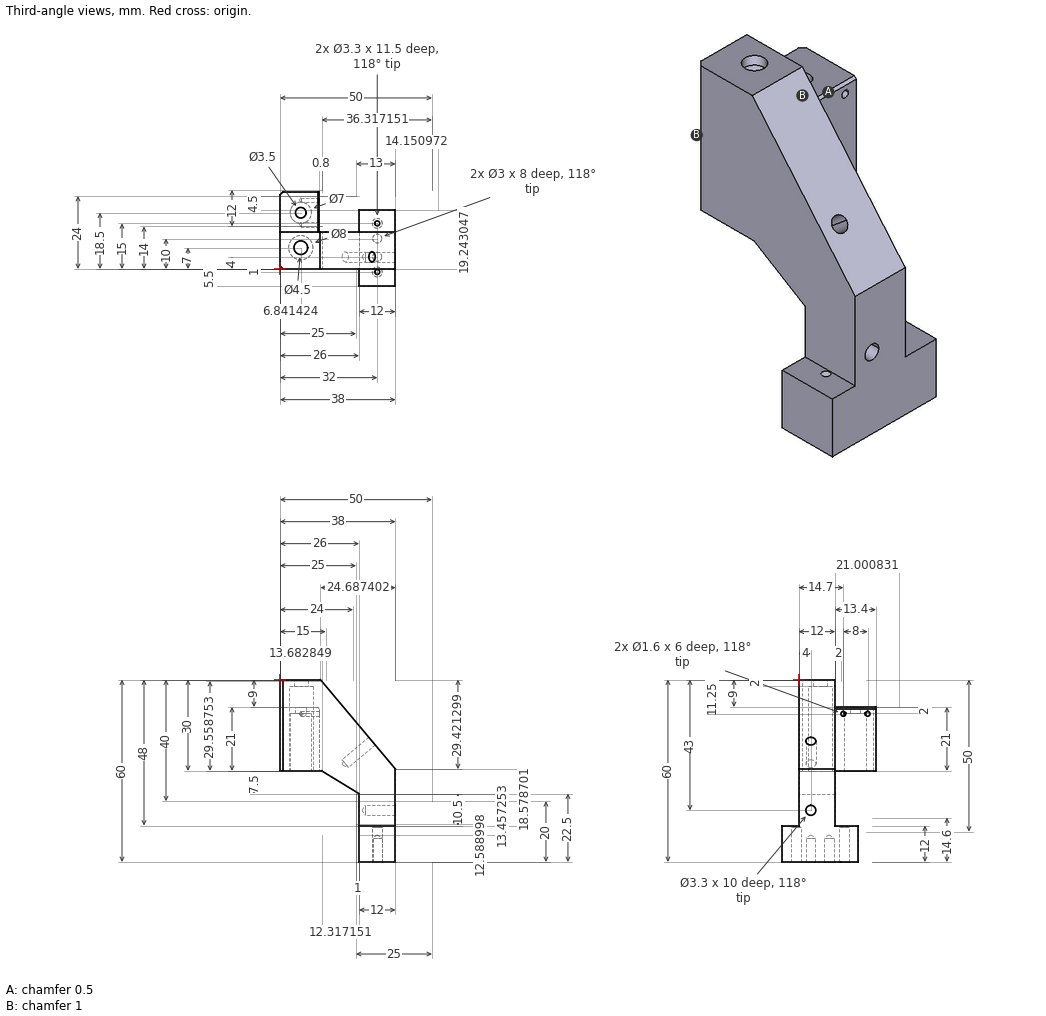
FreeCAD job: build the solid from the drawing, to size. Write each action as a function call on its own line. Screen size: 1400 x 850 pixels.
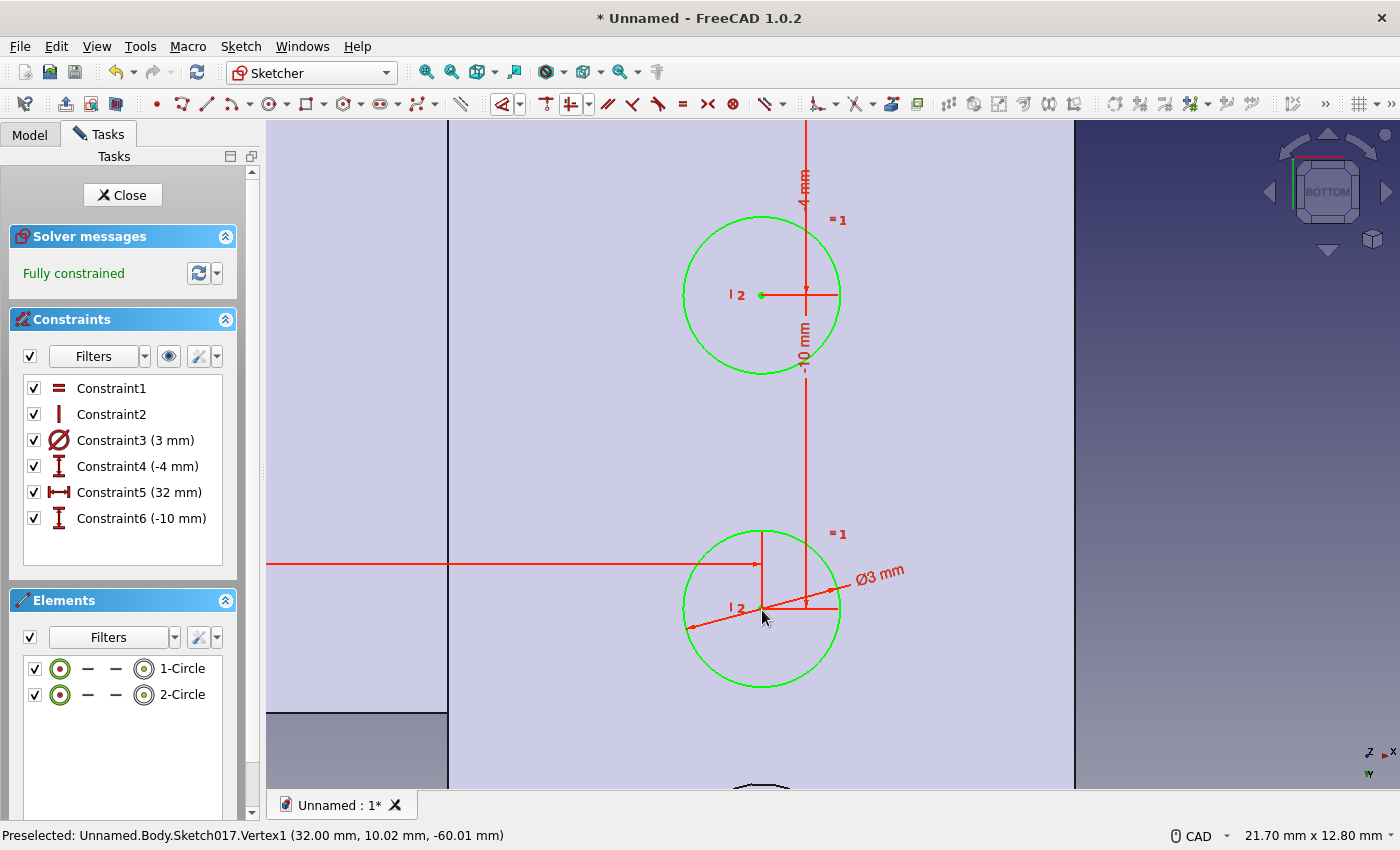
click(123, 195)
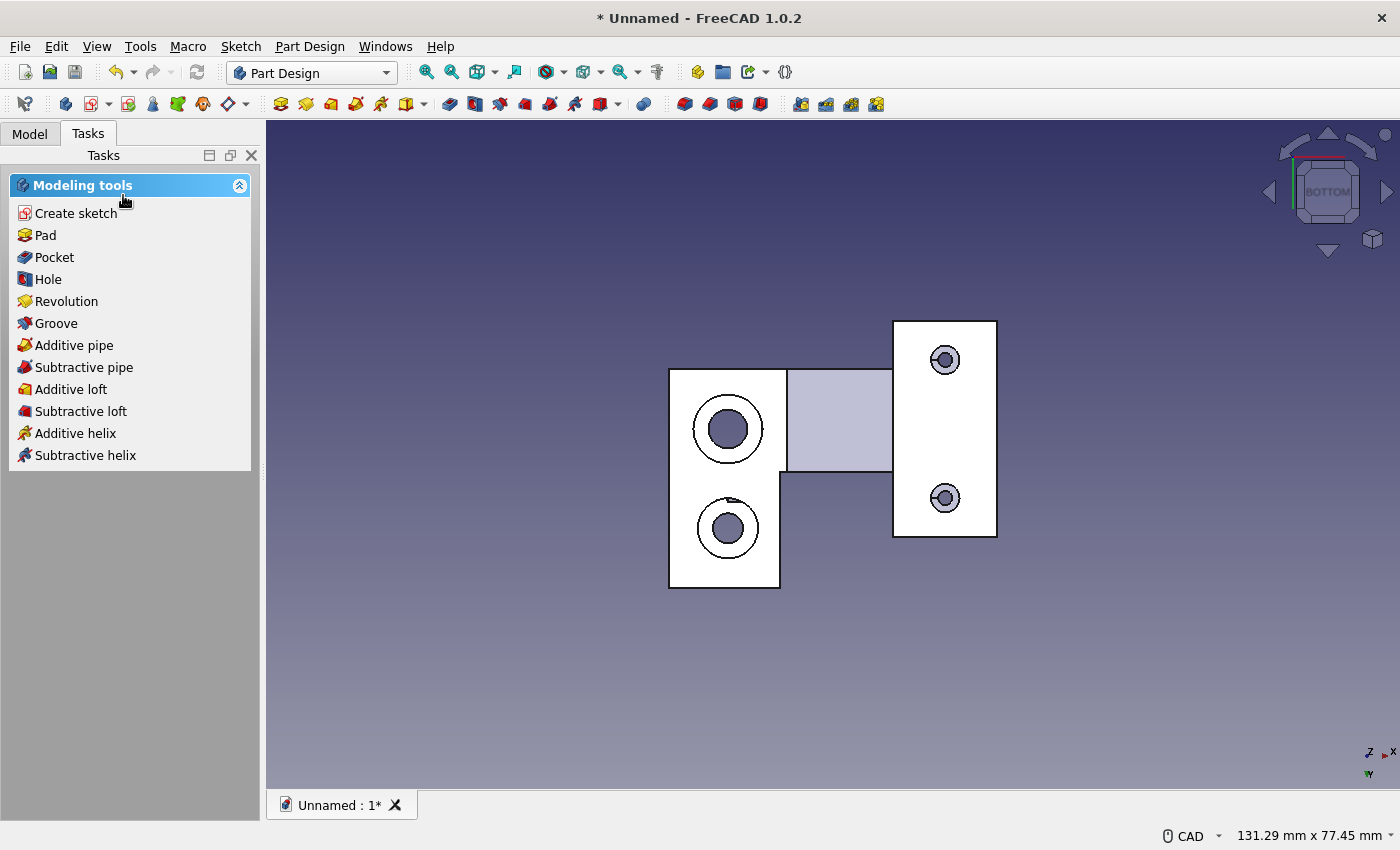
click(475, 104)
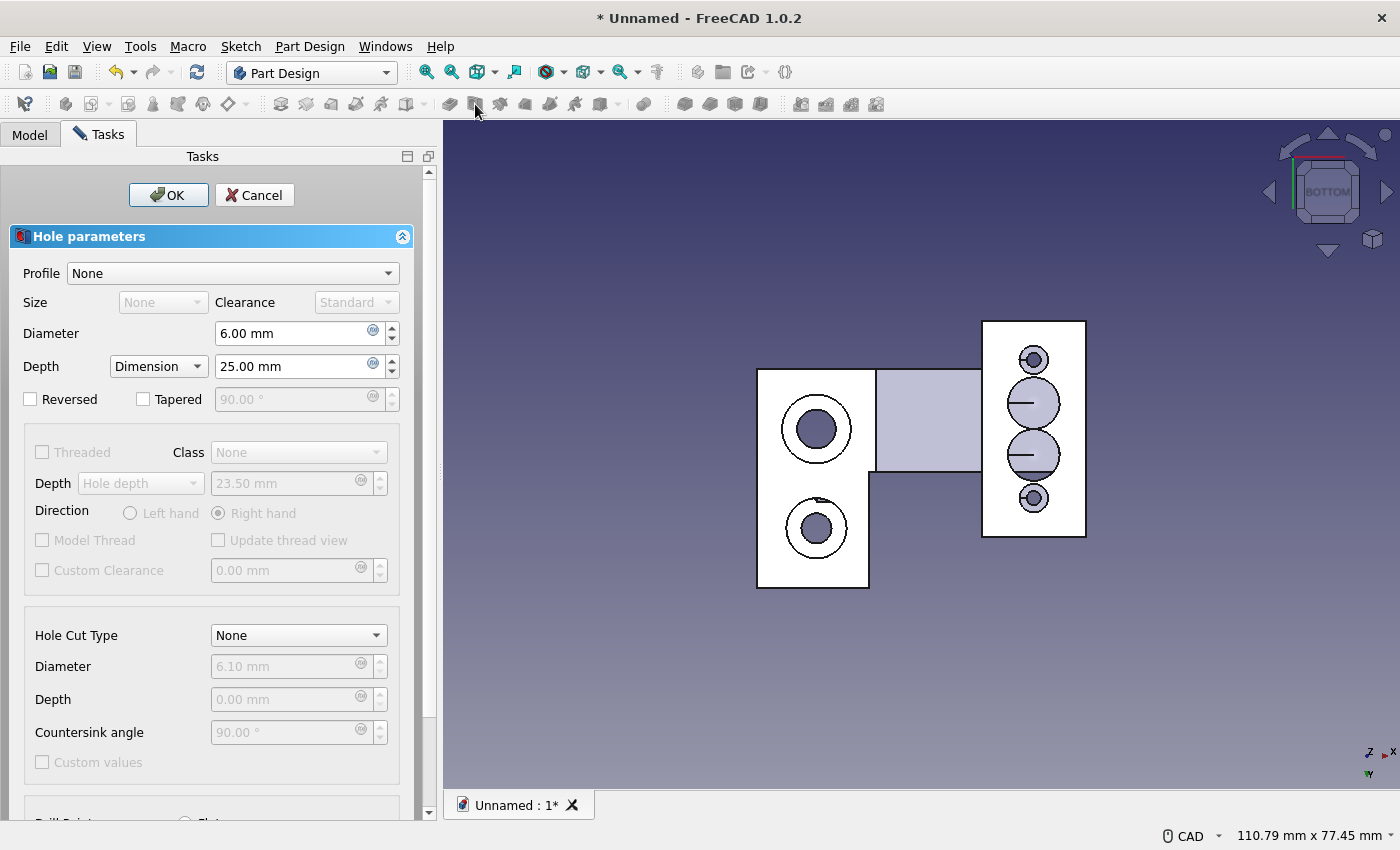
triple_click(300, 334)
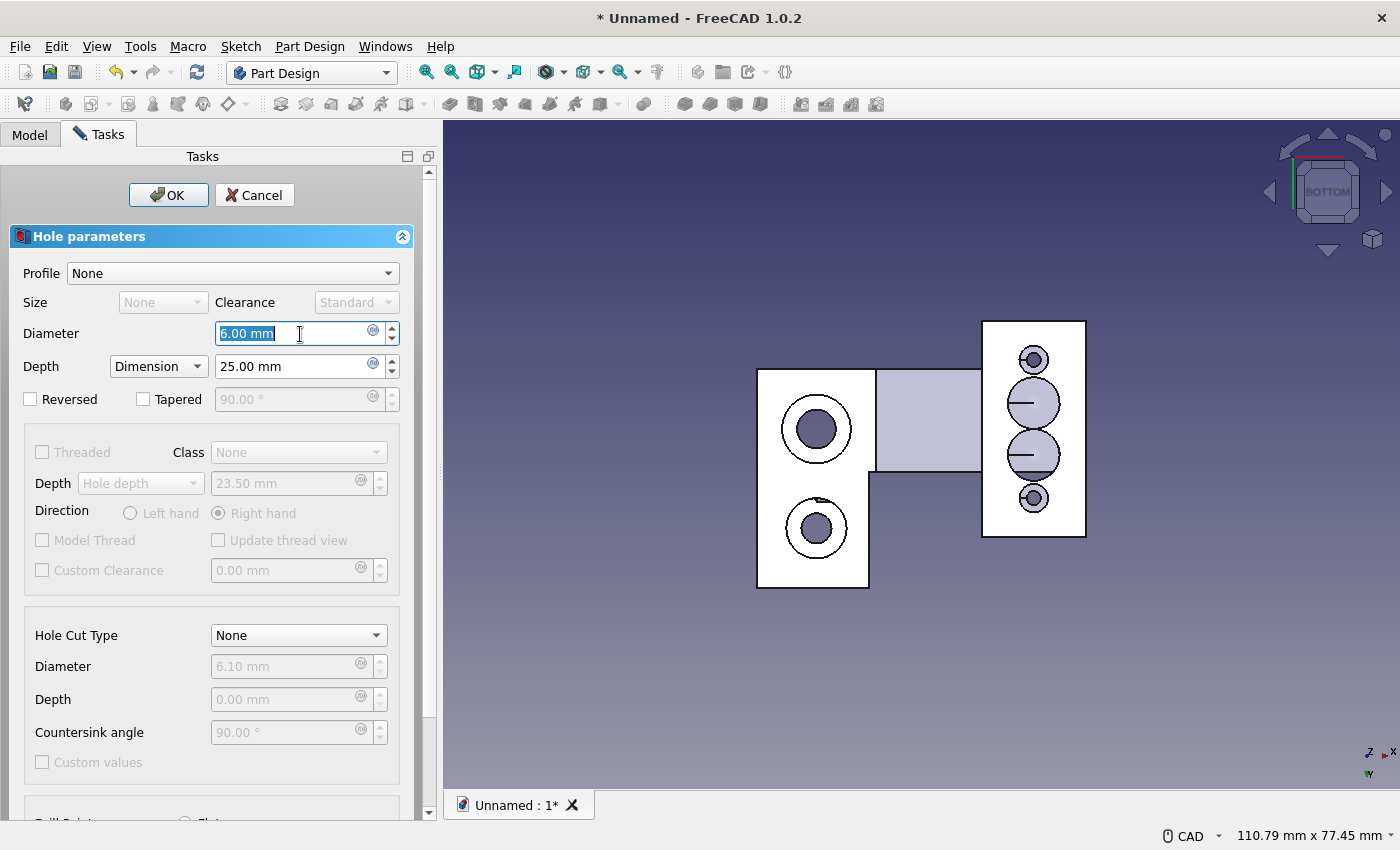
text(3)
key(Tab)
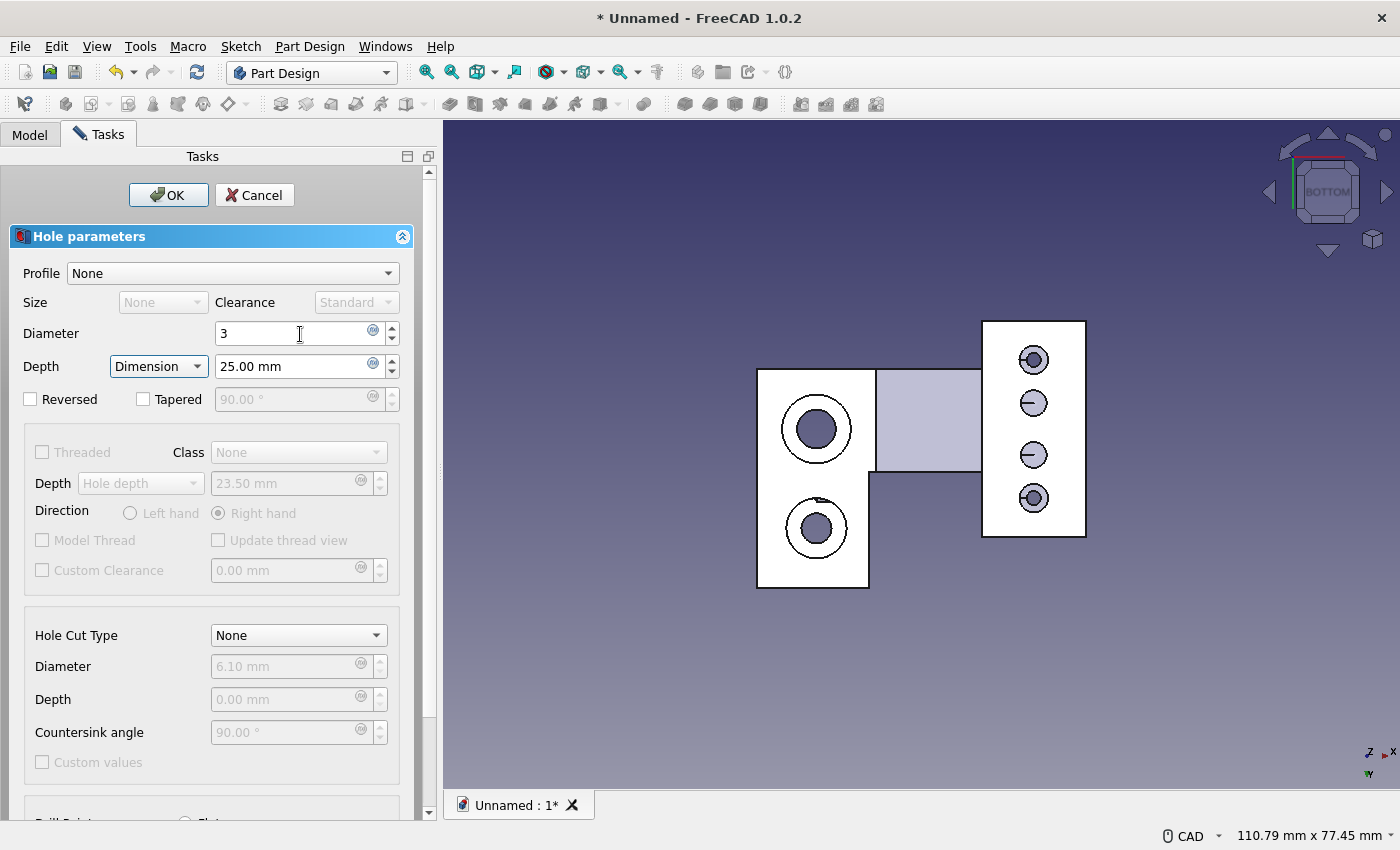
triple_click(300, 366)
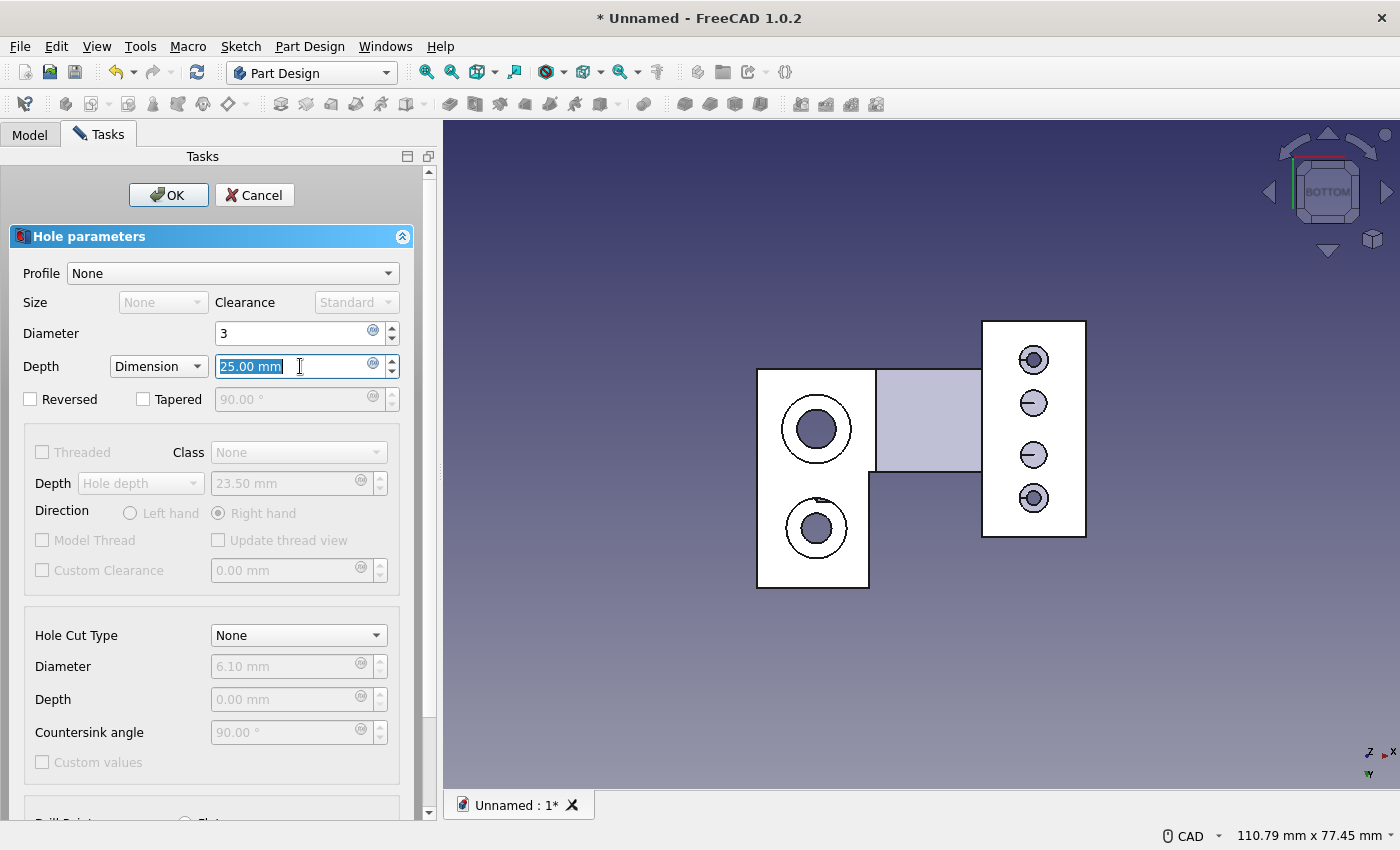
text(8)
key(Tab)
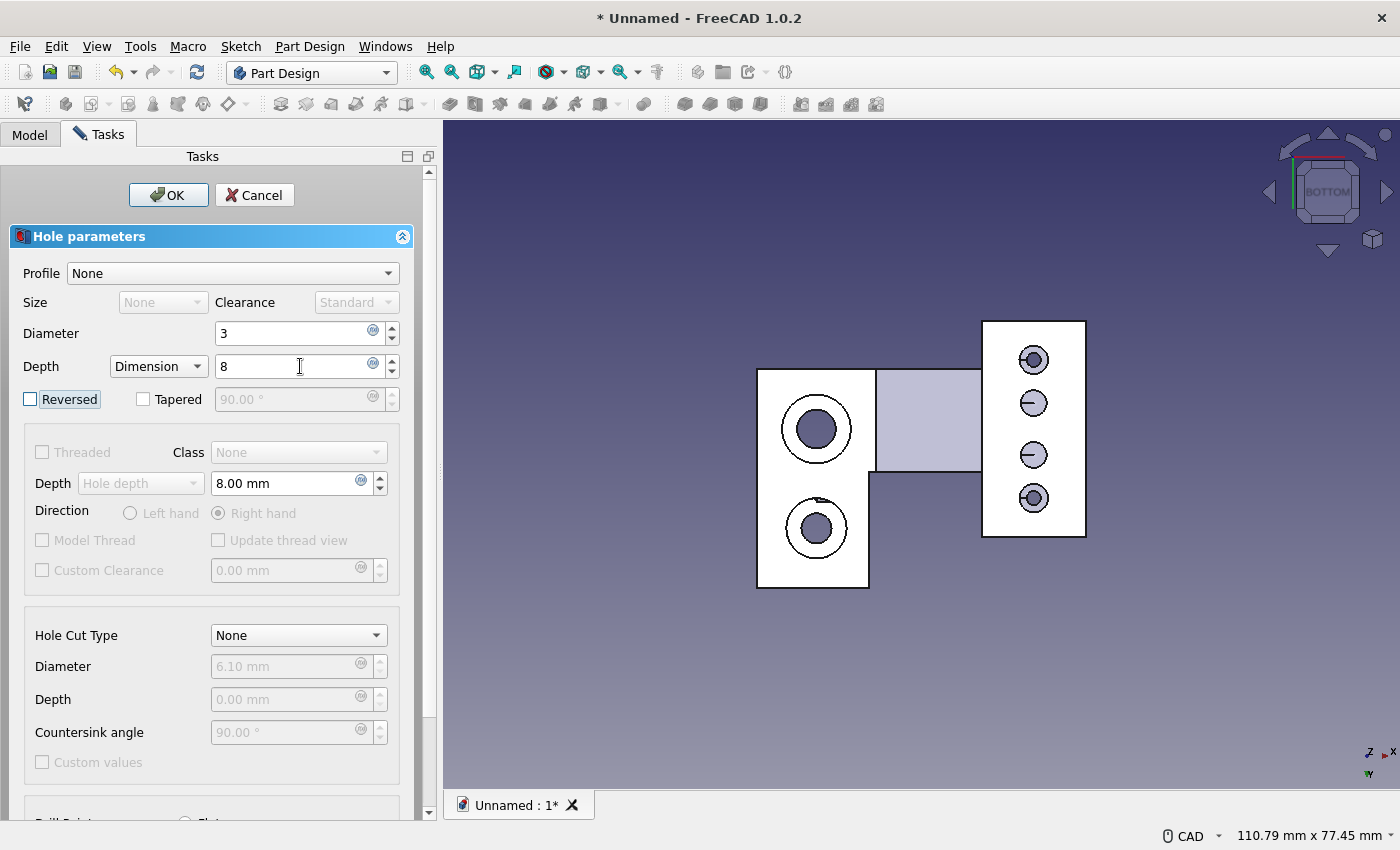
click(169, 195)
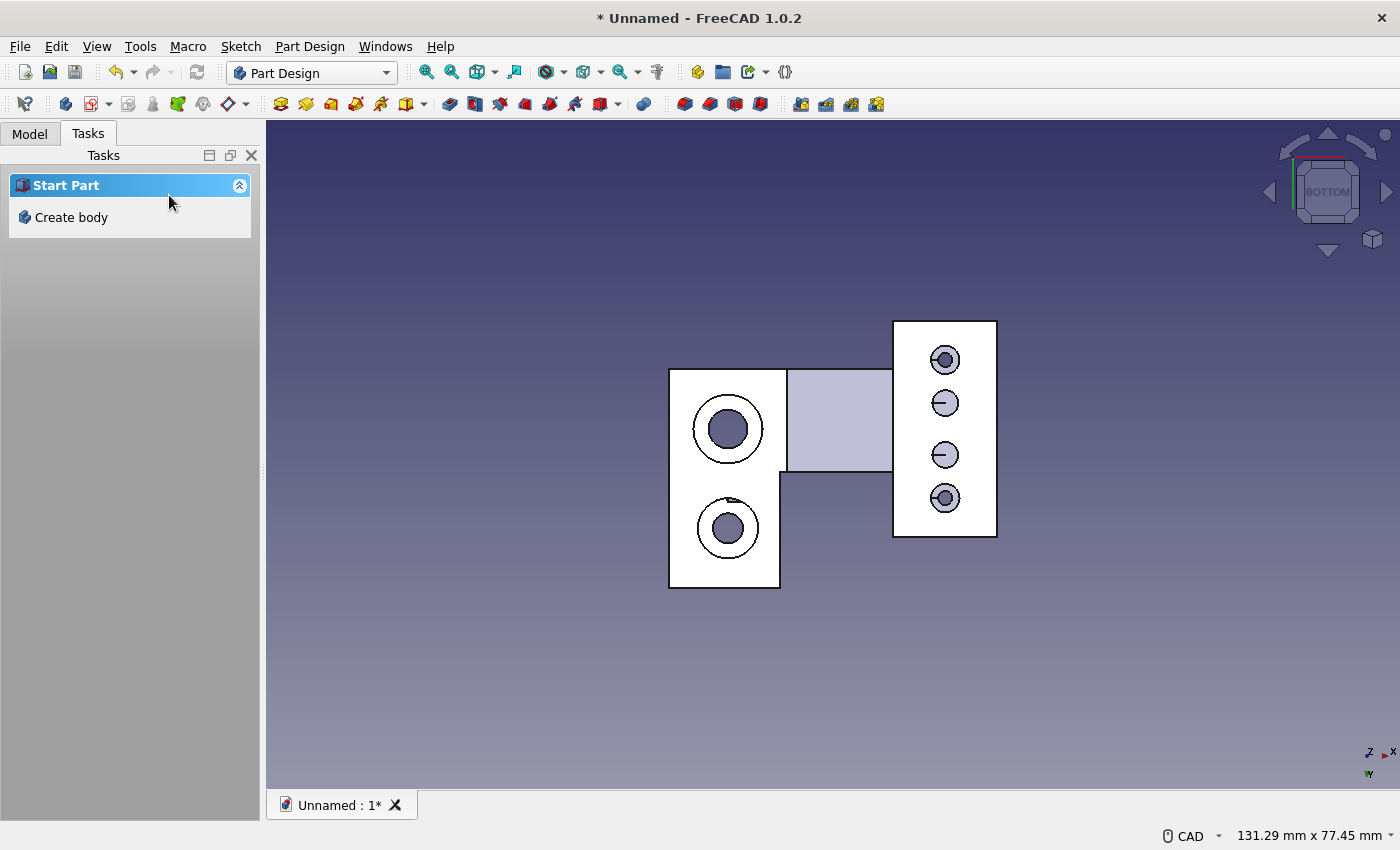
click(427, 72)